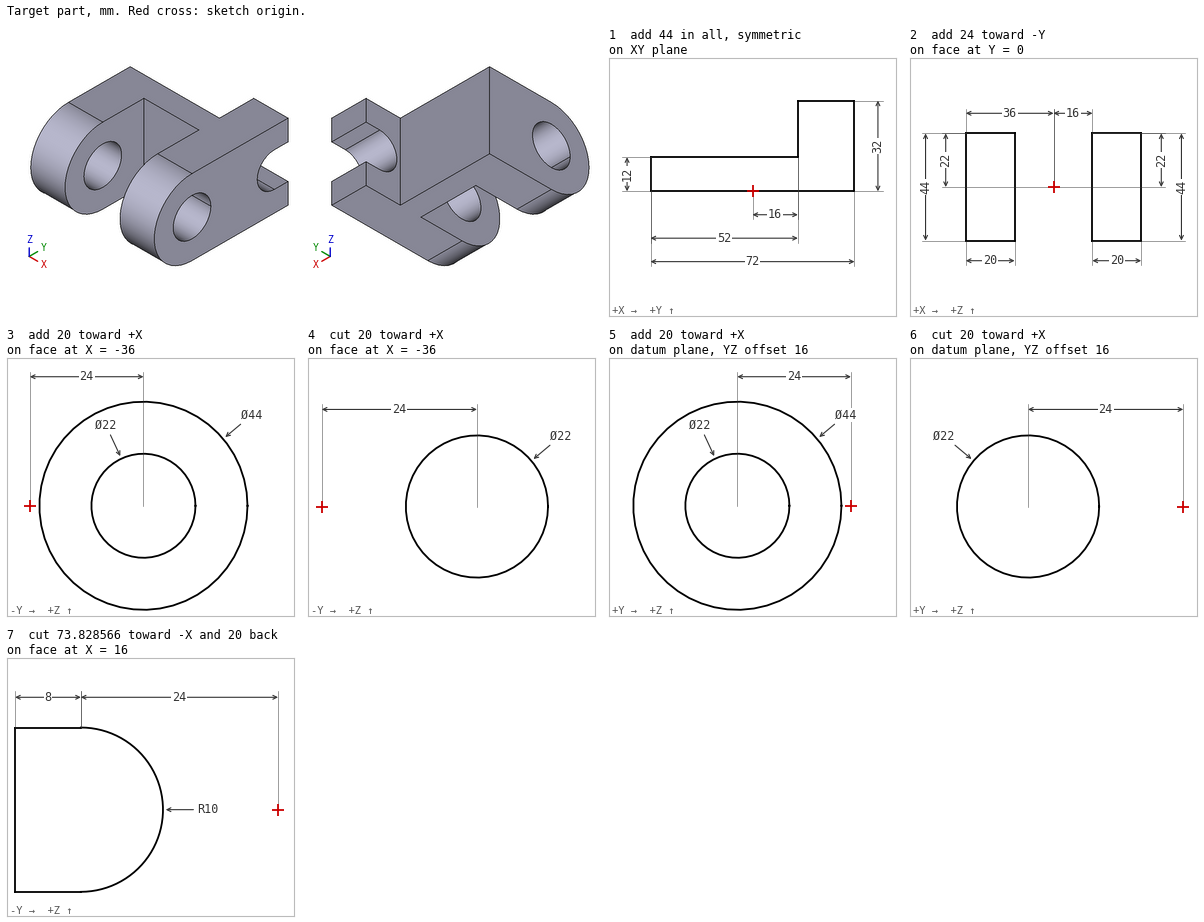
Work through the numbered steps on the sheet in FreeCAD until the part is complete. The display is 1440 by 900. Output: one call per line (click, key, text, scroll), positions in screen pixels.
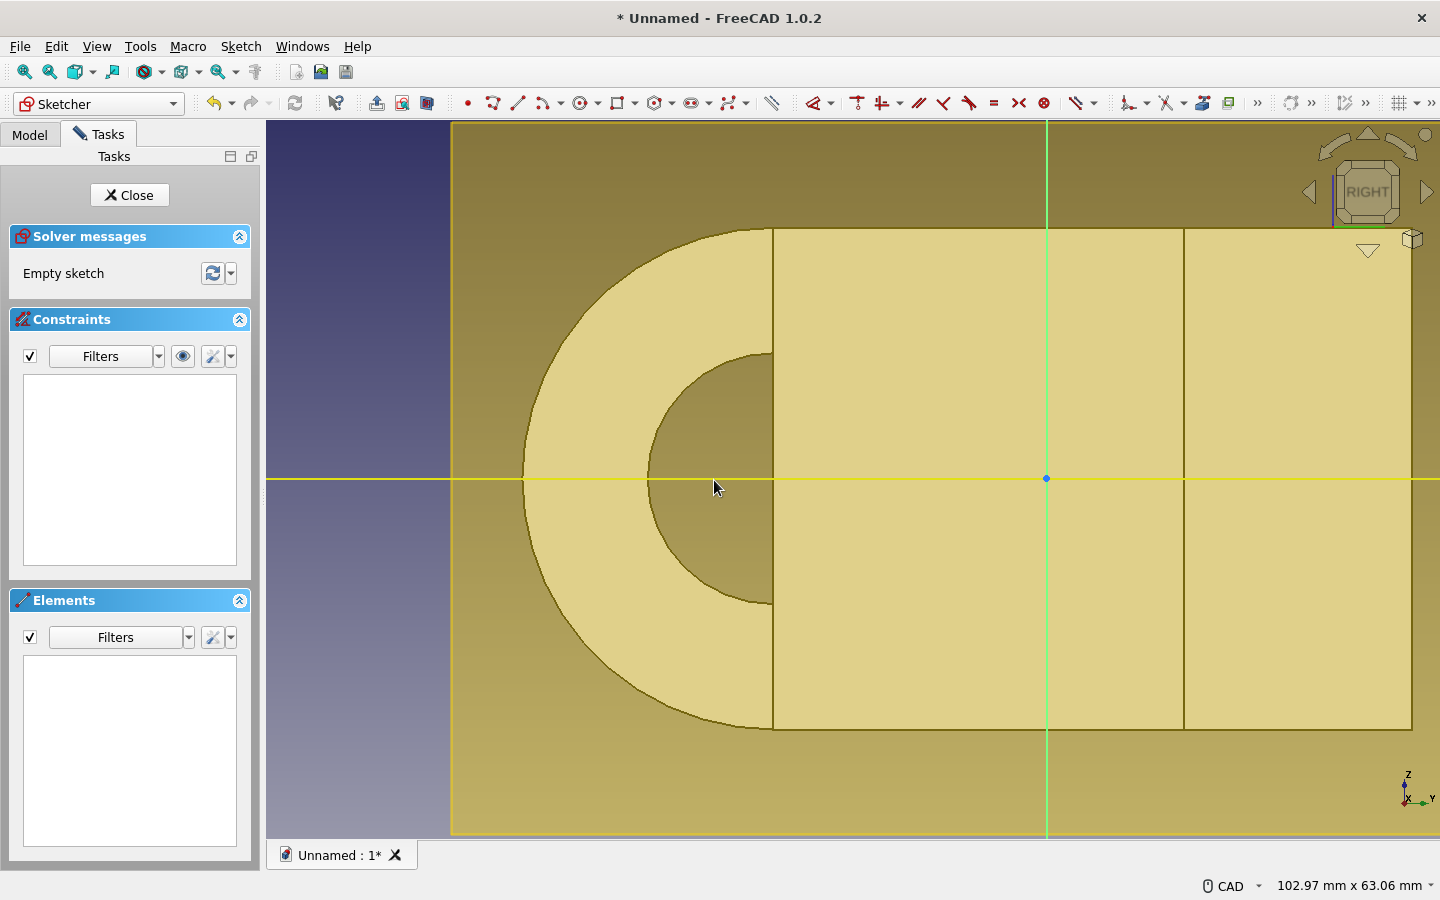
click(580, 104)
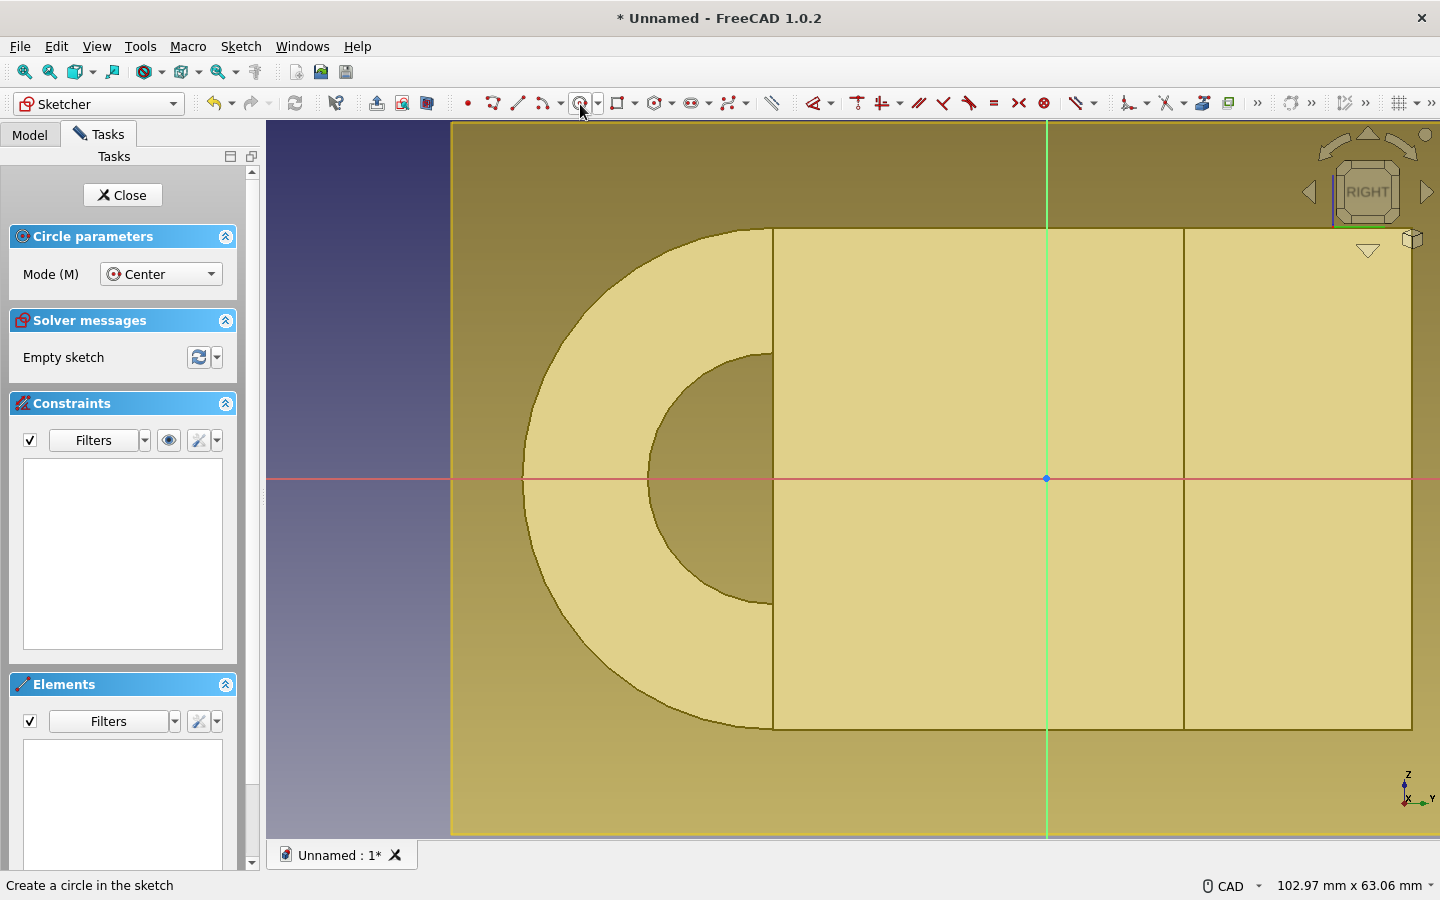
click(773, 479)
click(951, 301)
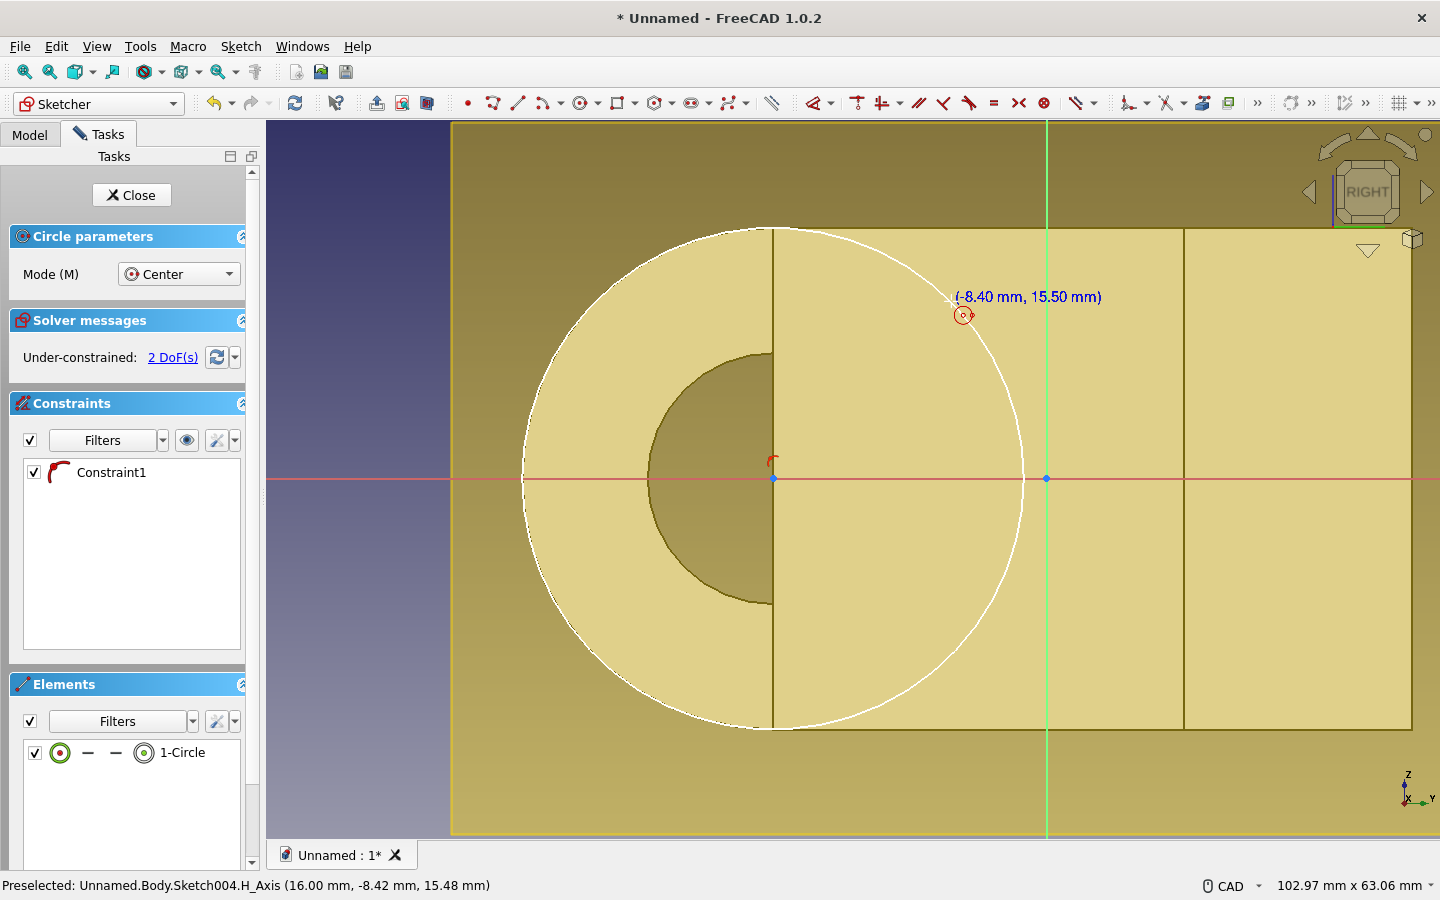
click(773, 479)
click(862, 390)
key(Escape)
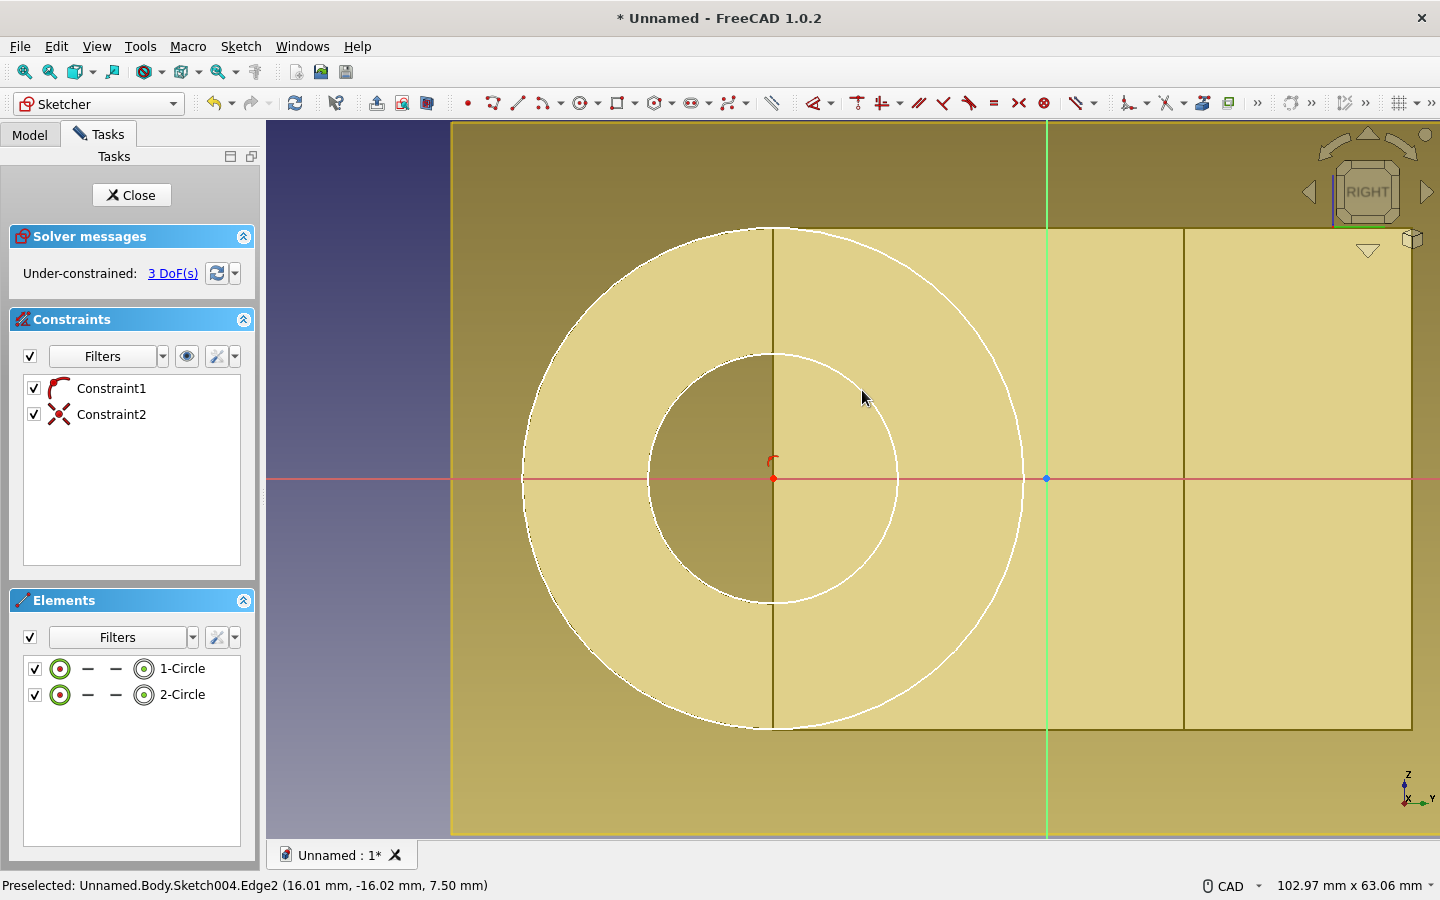
click(812, 104)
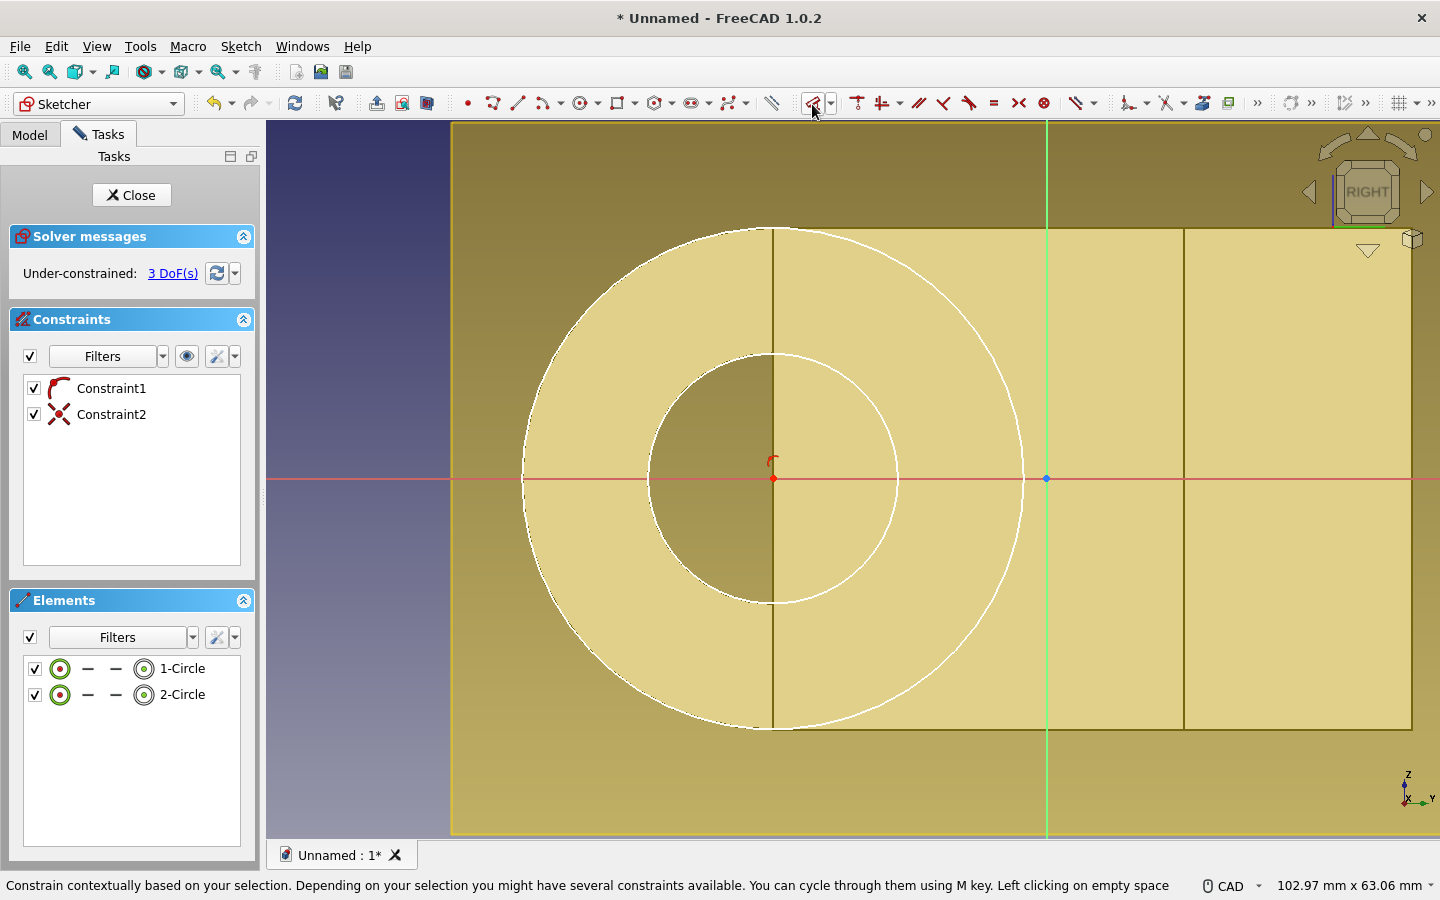
click(950, 301)
click(973, 278)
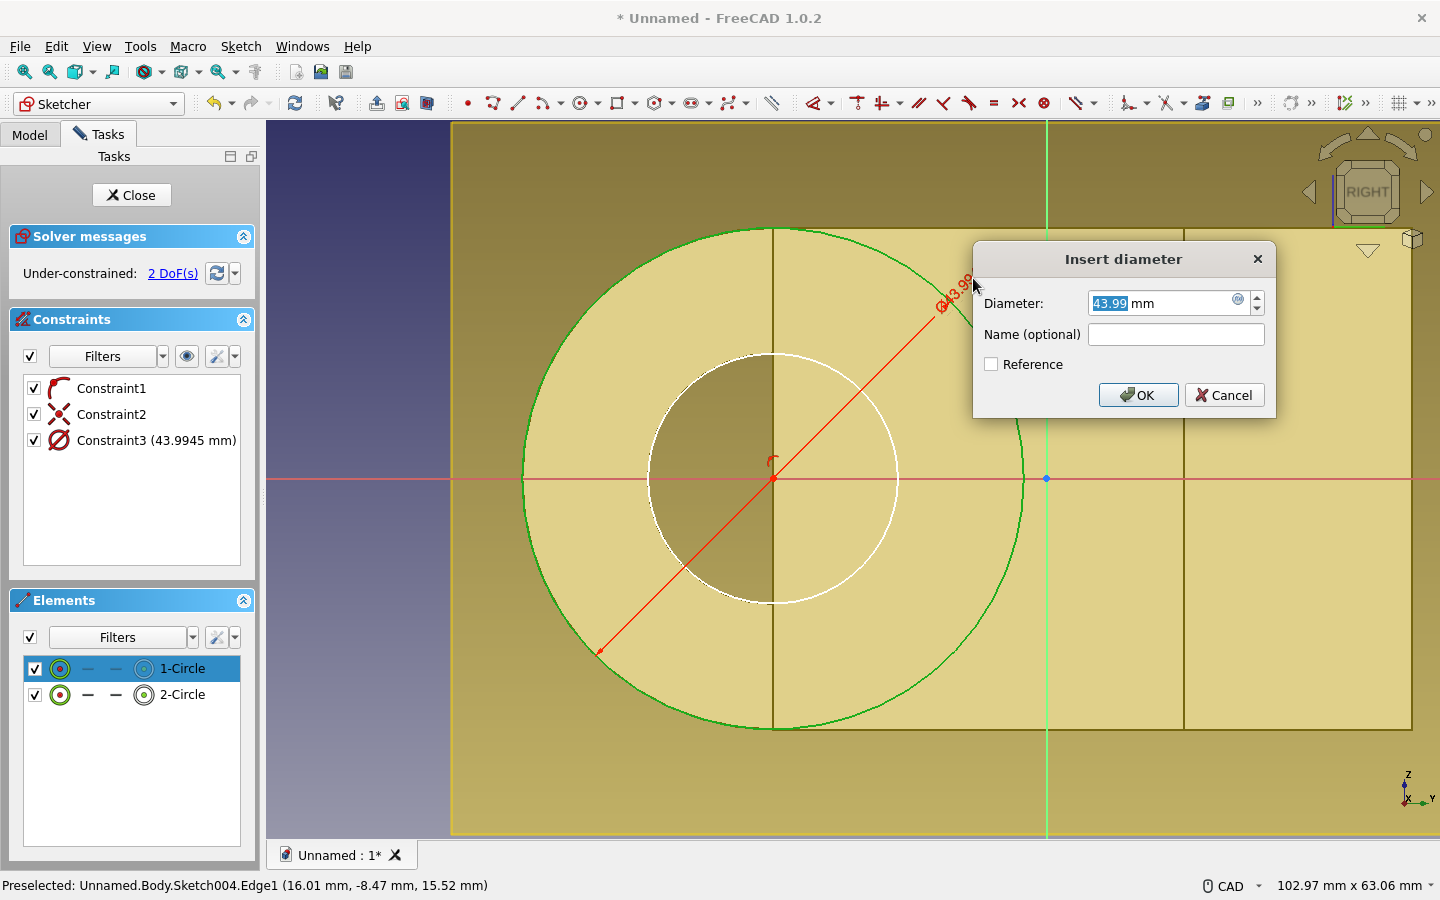
text(44)
key(Return)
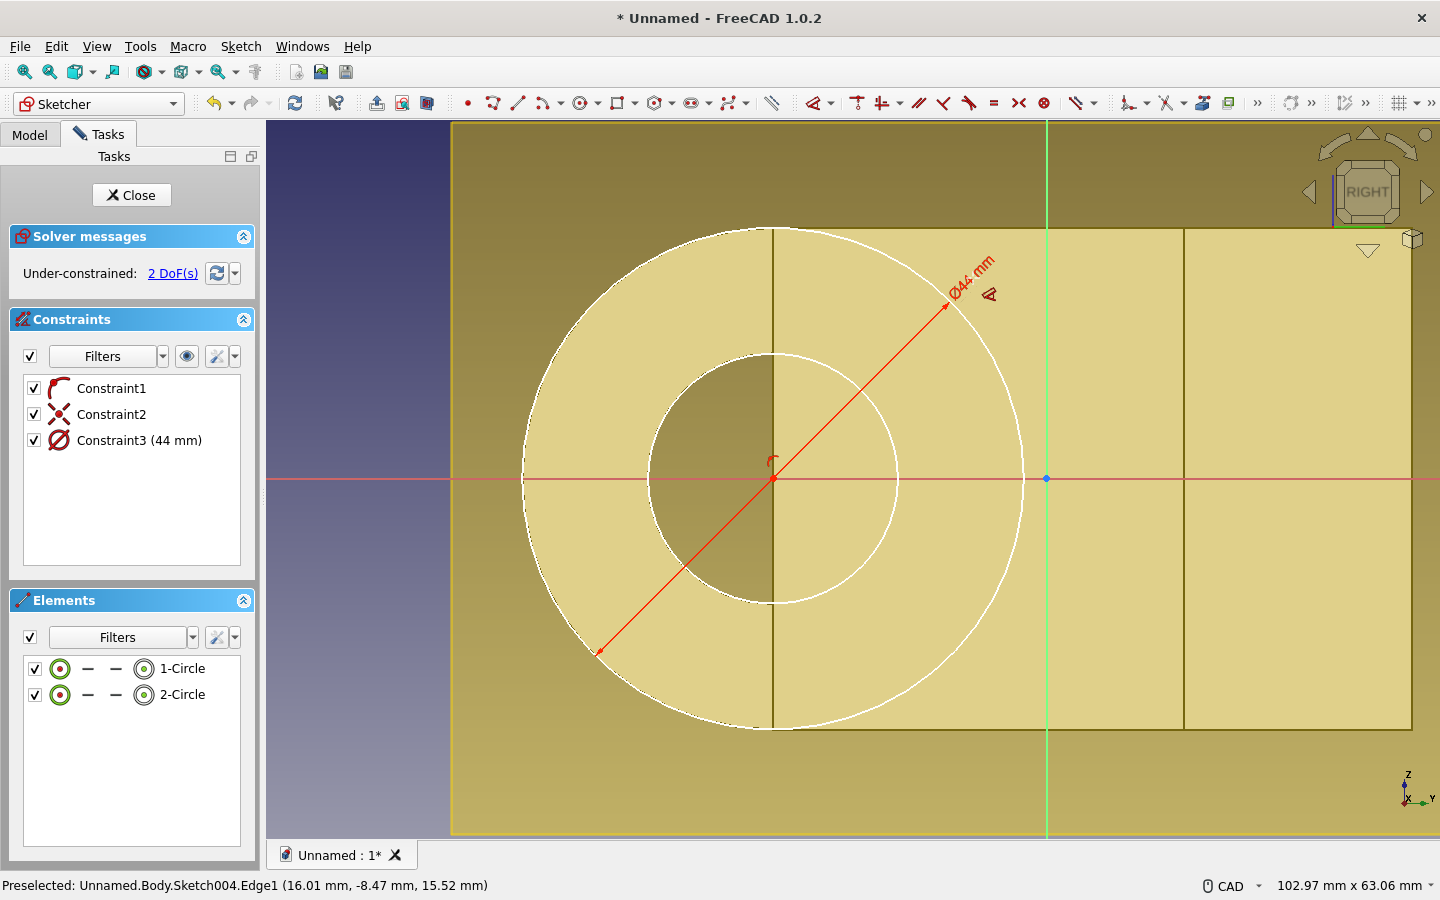
click(861, 390)
click(884, 367)